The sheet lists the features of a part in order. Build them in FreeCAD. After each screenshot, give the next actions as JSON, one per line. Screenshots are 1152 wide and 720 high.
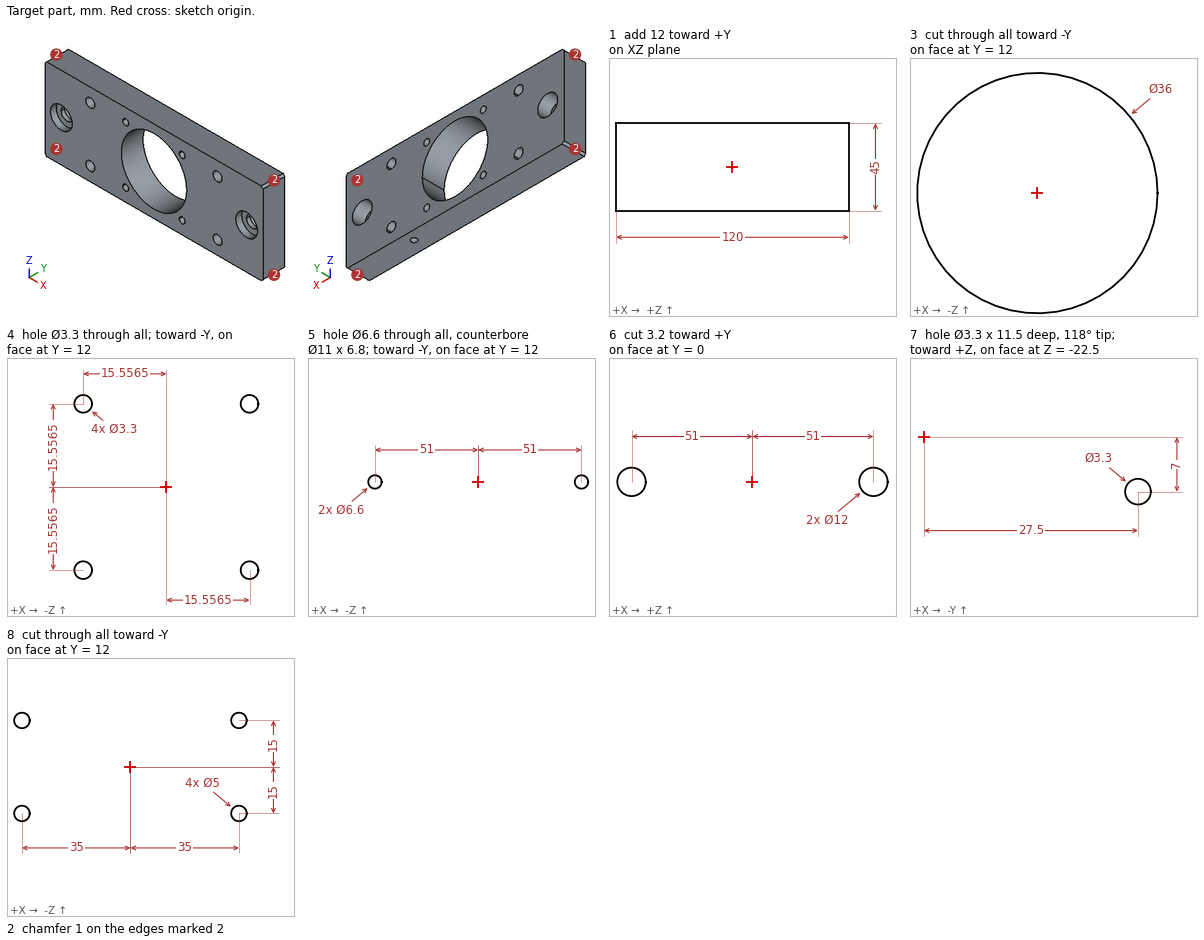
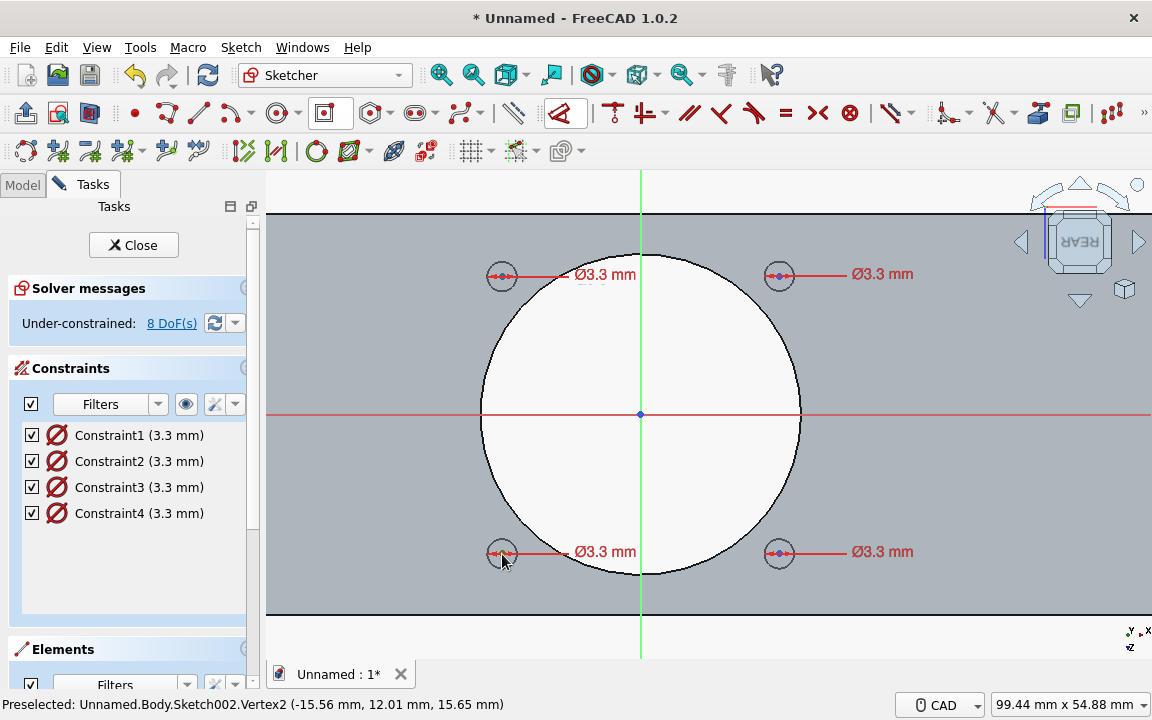
{"action": "left_click", "coordinate": [668, 114]}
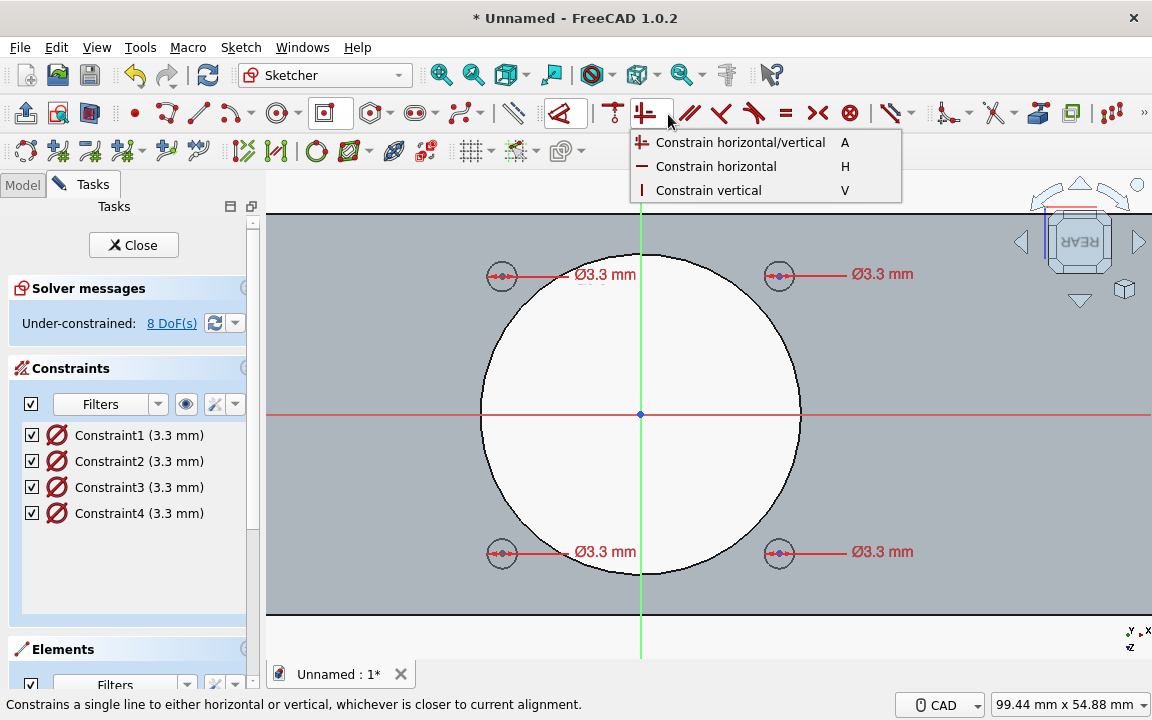
{"action": "left_click", "coordinate": [766, 190]}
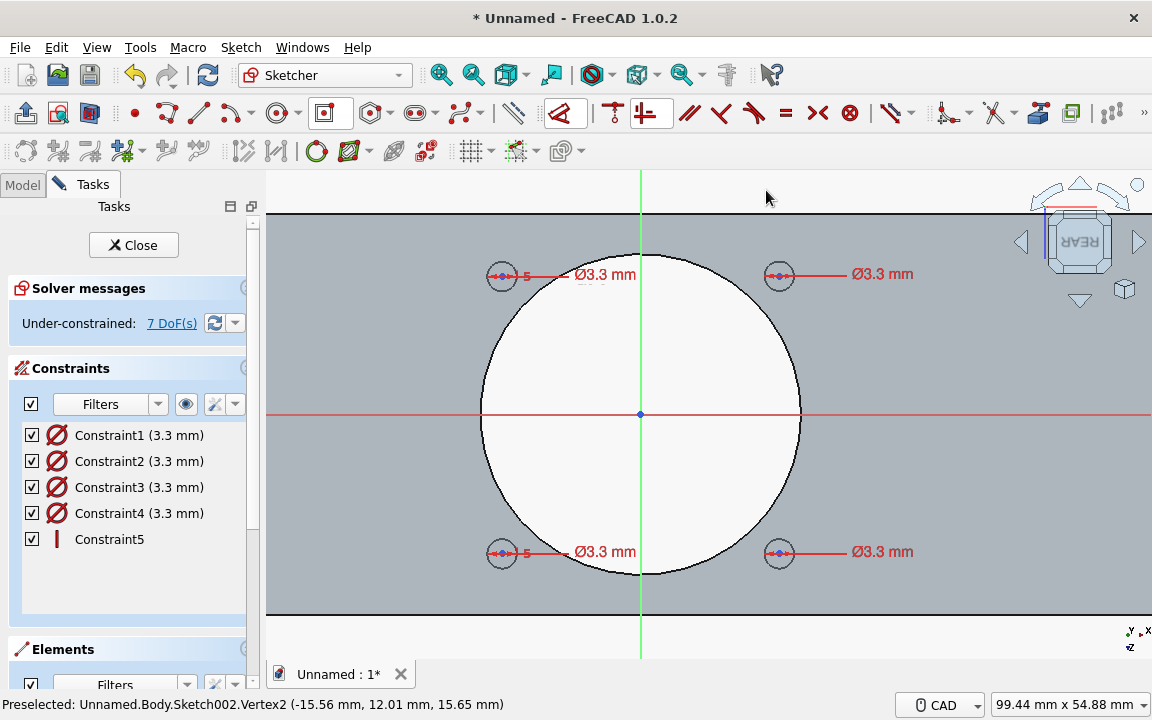
{"action": "left_click", "coordinate": [502, 554]}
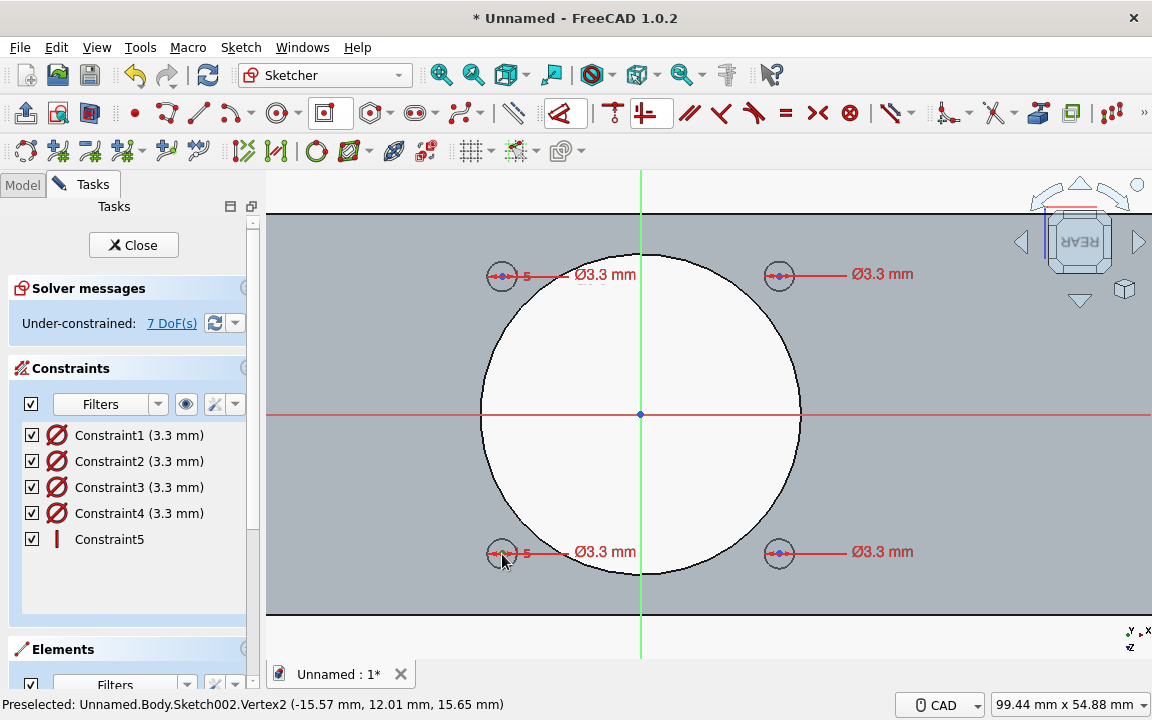
{"action": "left_click", "coordinate": [779, 554]}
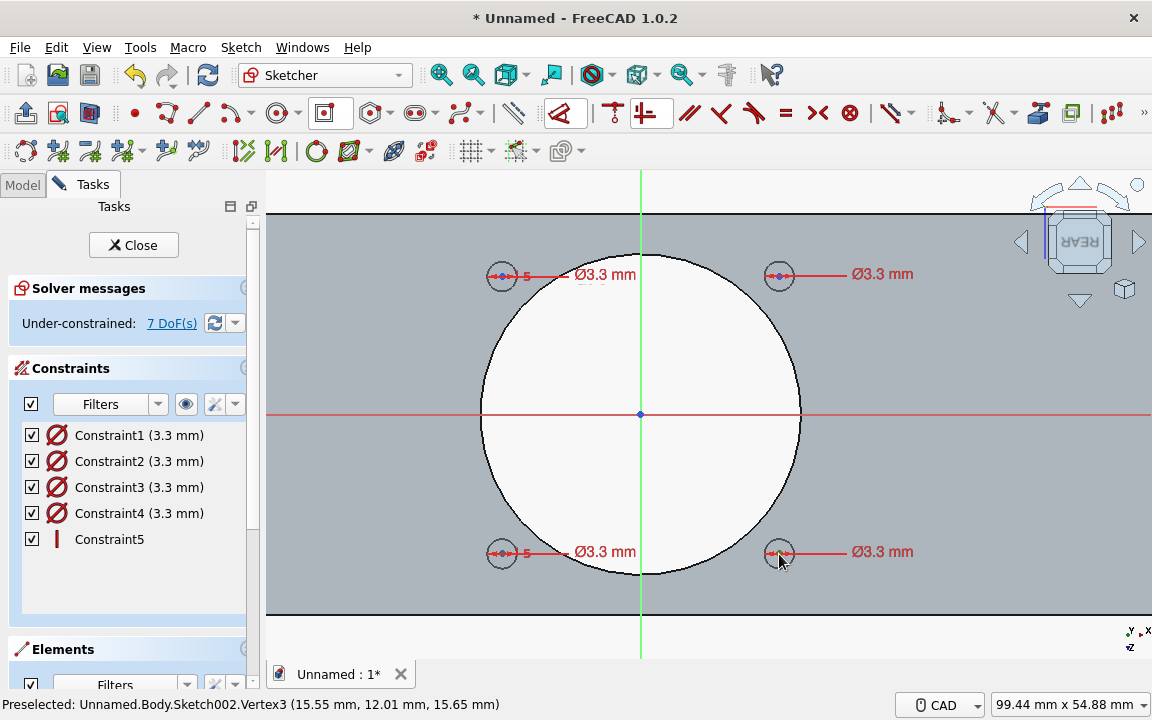
{"action": "left_click", "coordinate": [668, 114]}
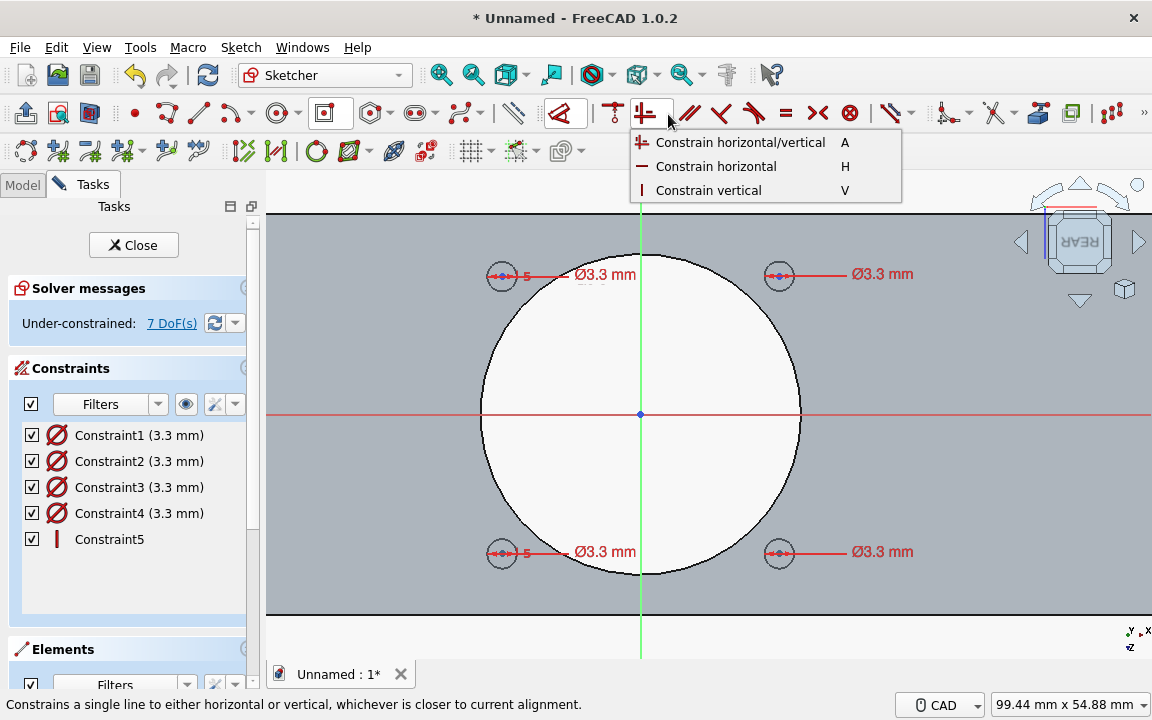
{"action": "left_click", "coordinate": [766, 166]}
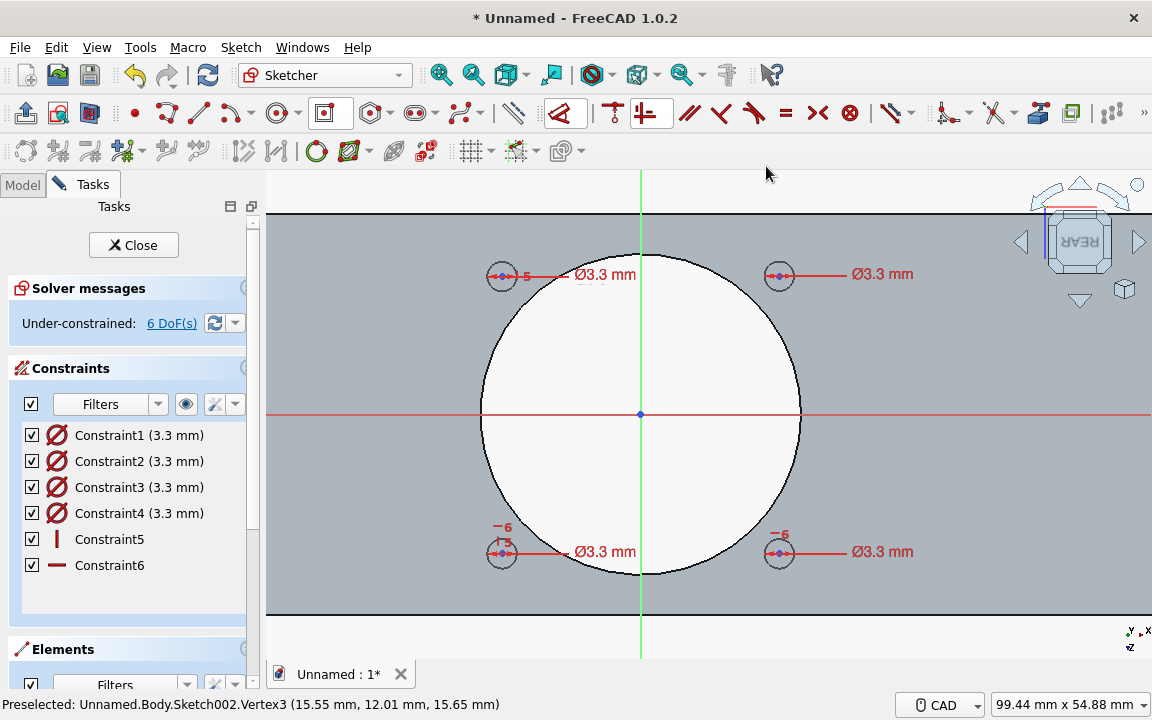
{"action": "left_click", "coordinate": [779, 554]}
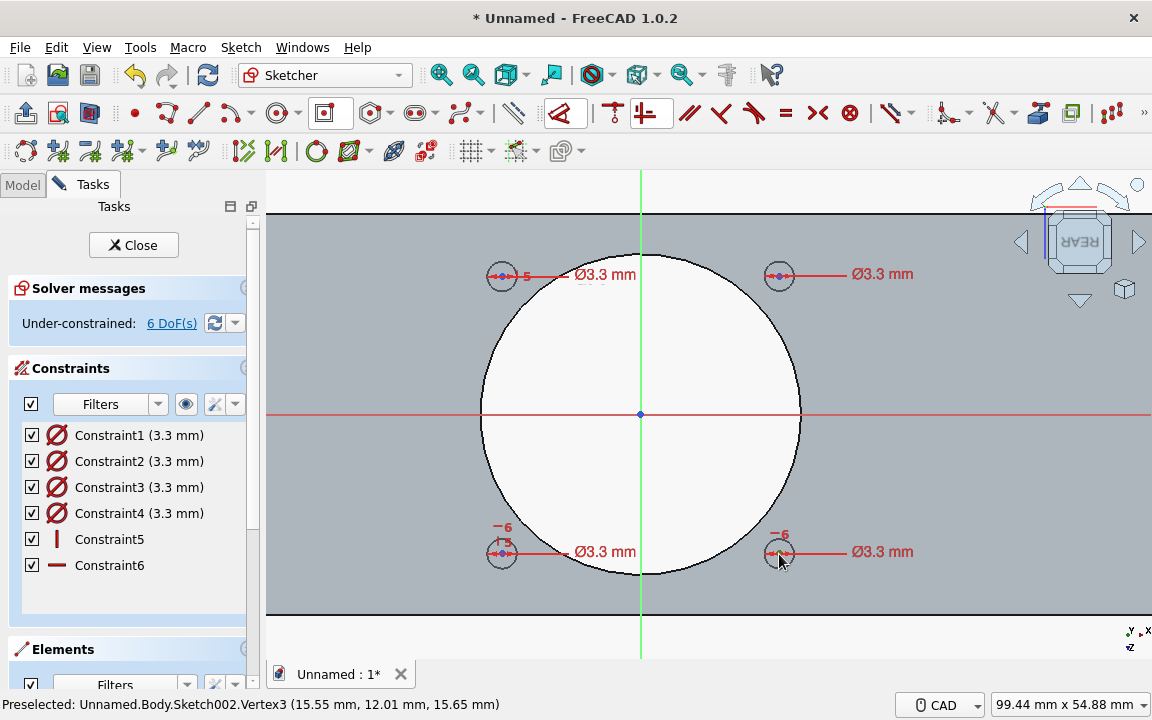
{"action": "left_click", "coordinate": [779, 276]}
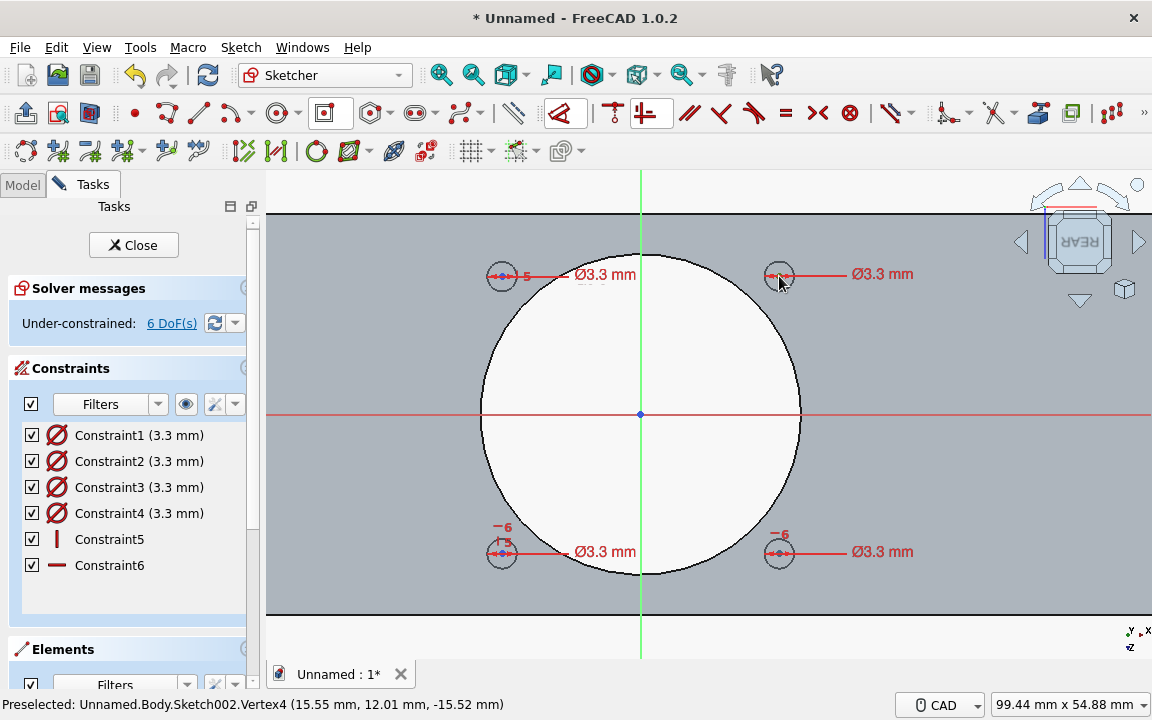
{"action": "key", "text": "v"}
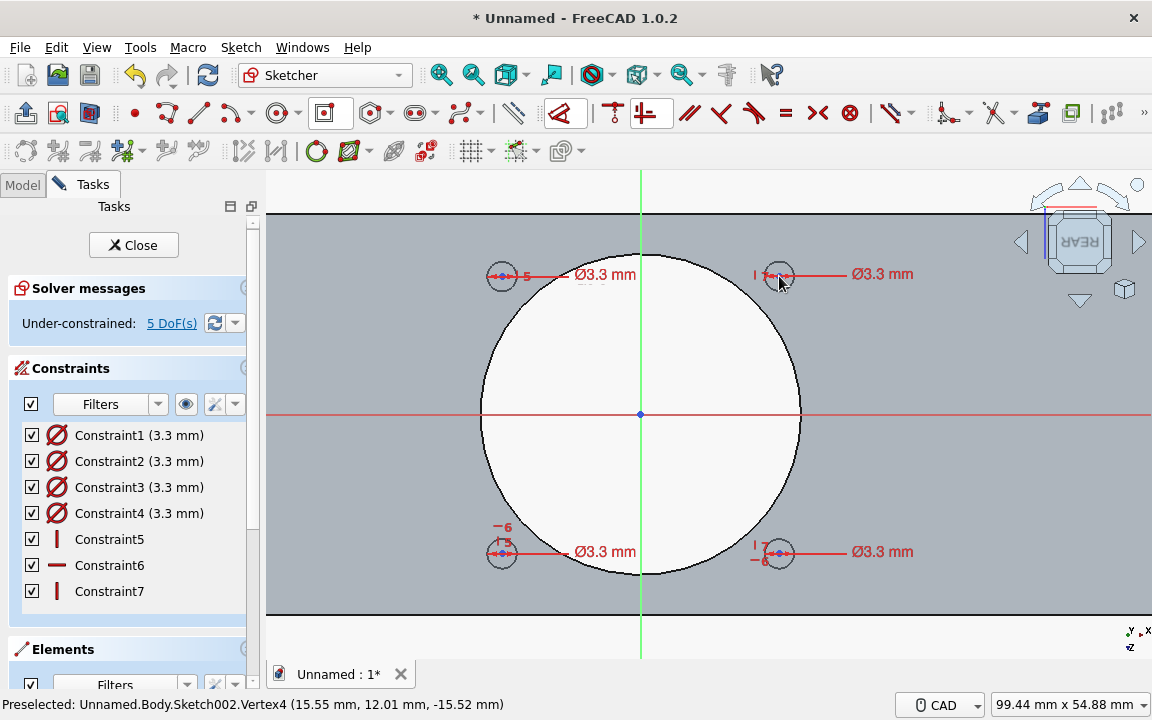
{"action": "left_click", "coordinate": [502, 277]}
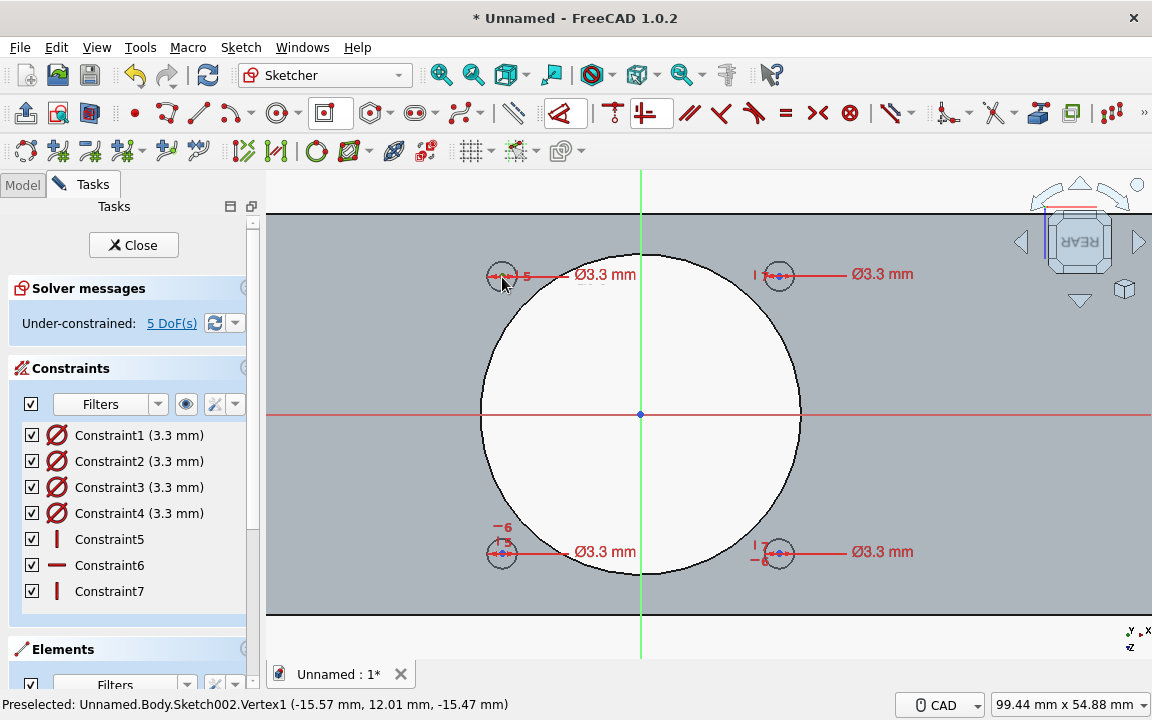
{"action": "left_click", "coordinate": [779, 276]}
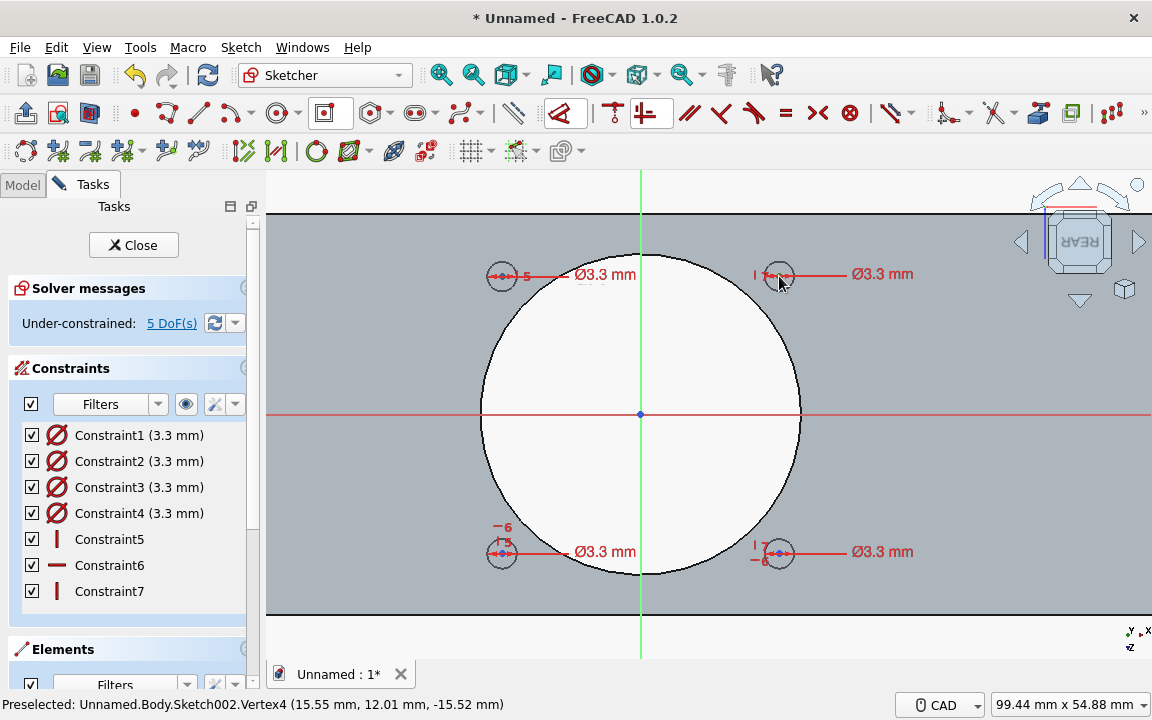
{"action": "left_click", "coordinate": [668, 114]}